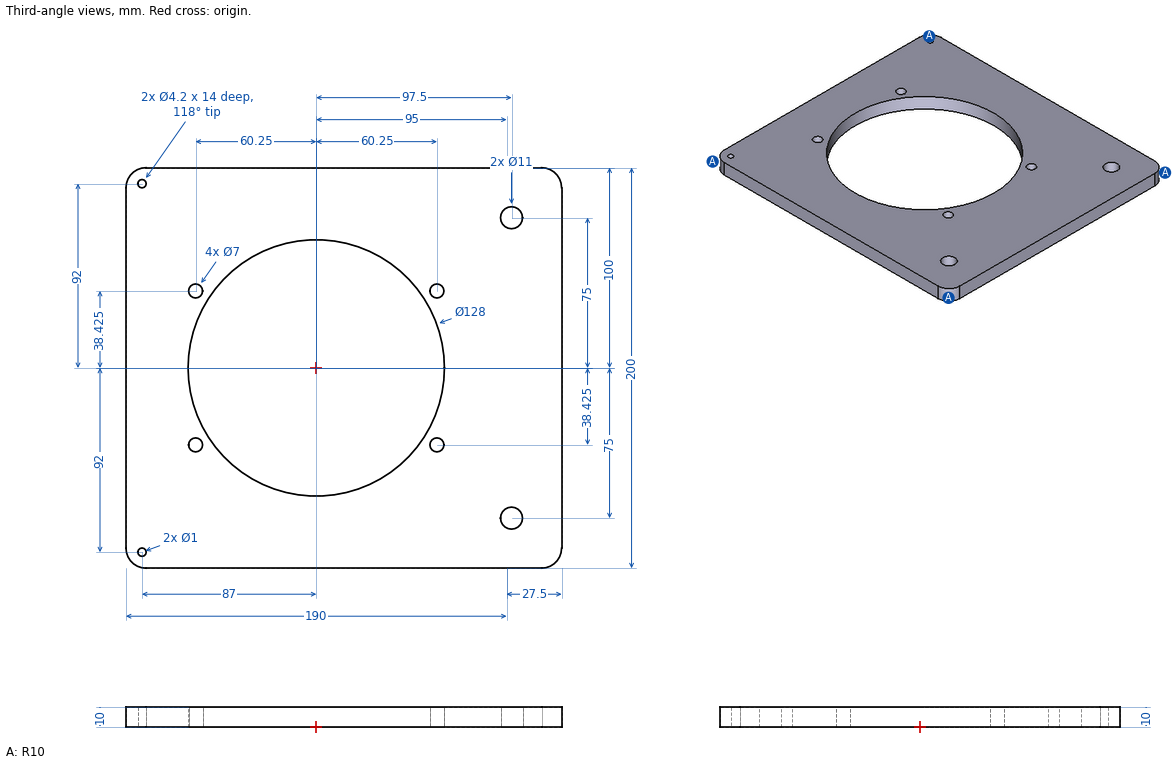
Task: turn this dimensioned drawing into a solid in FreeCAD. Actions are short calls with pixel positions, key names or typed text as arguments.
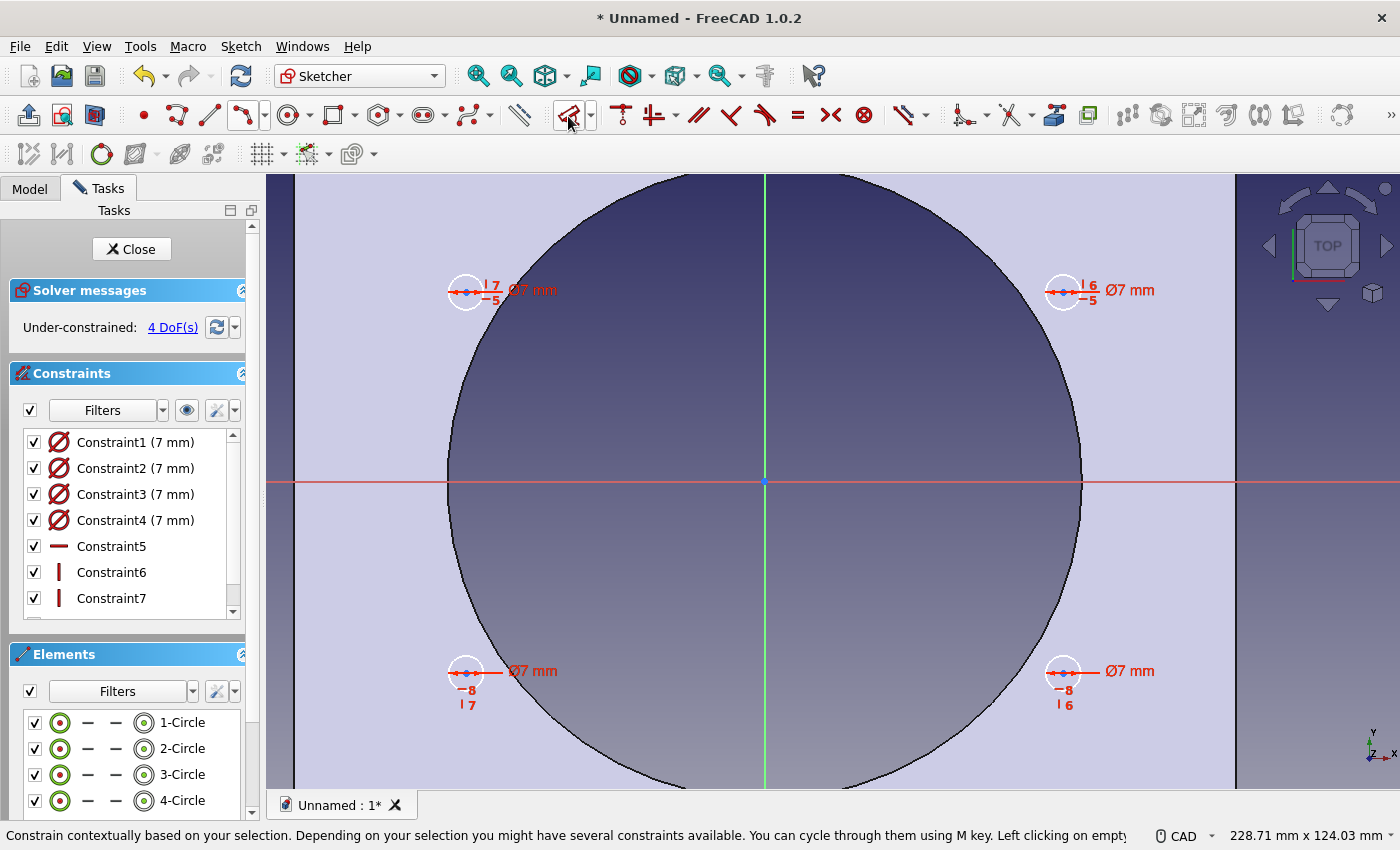
click(466, 292)
click(615, 258)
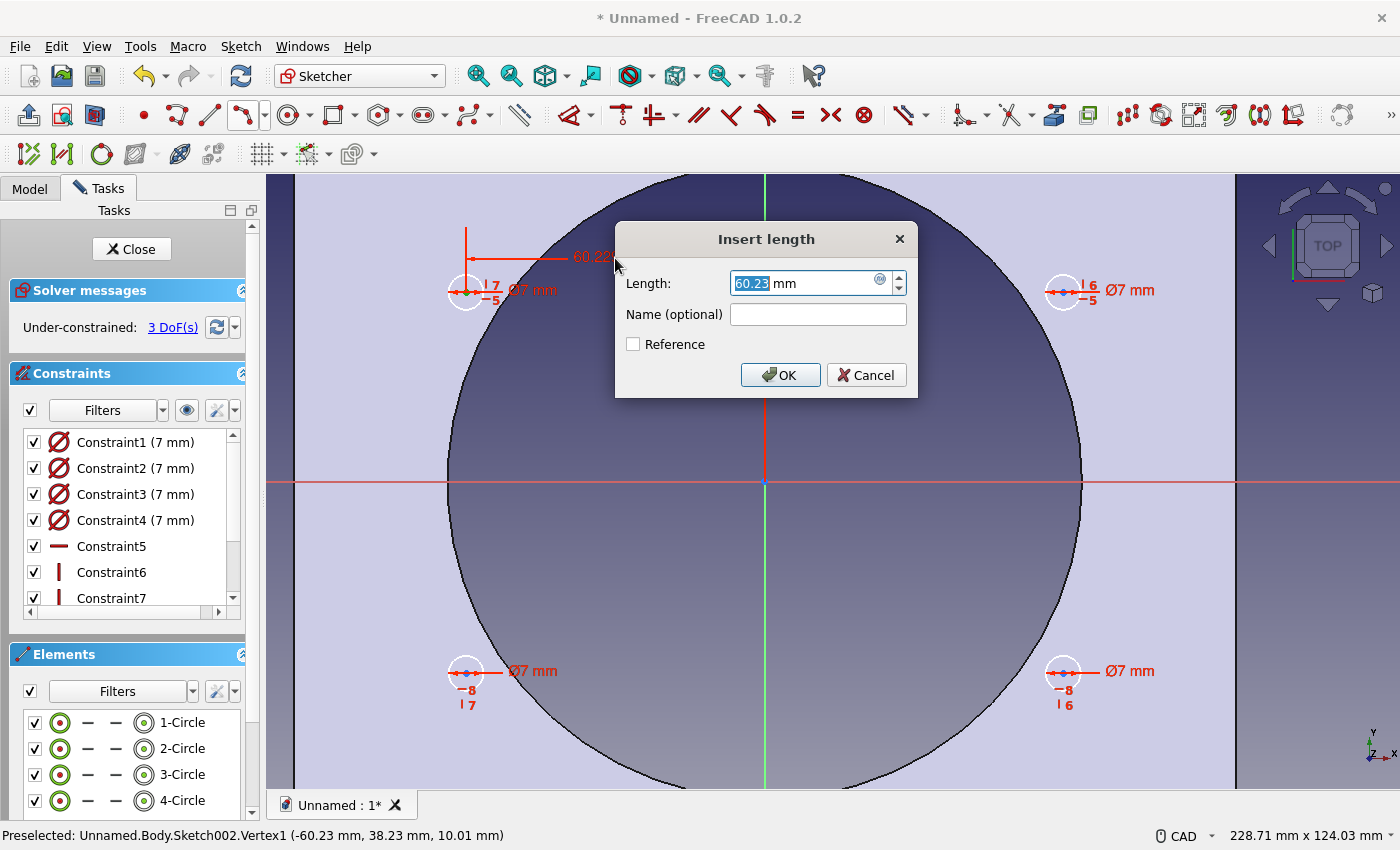
text(60.25)
key(Return)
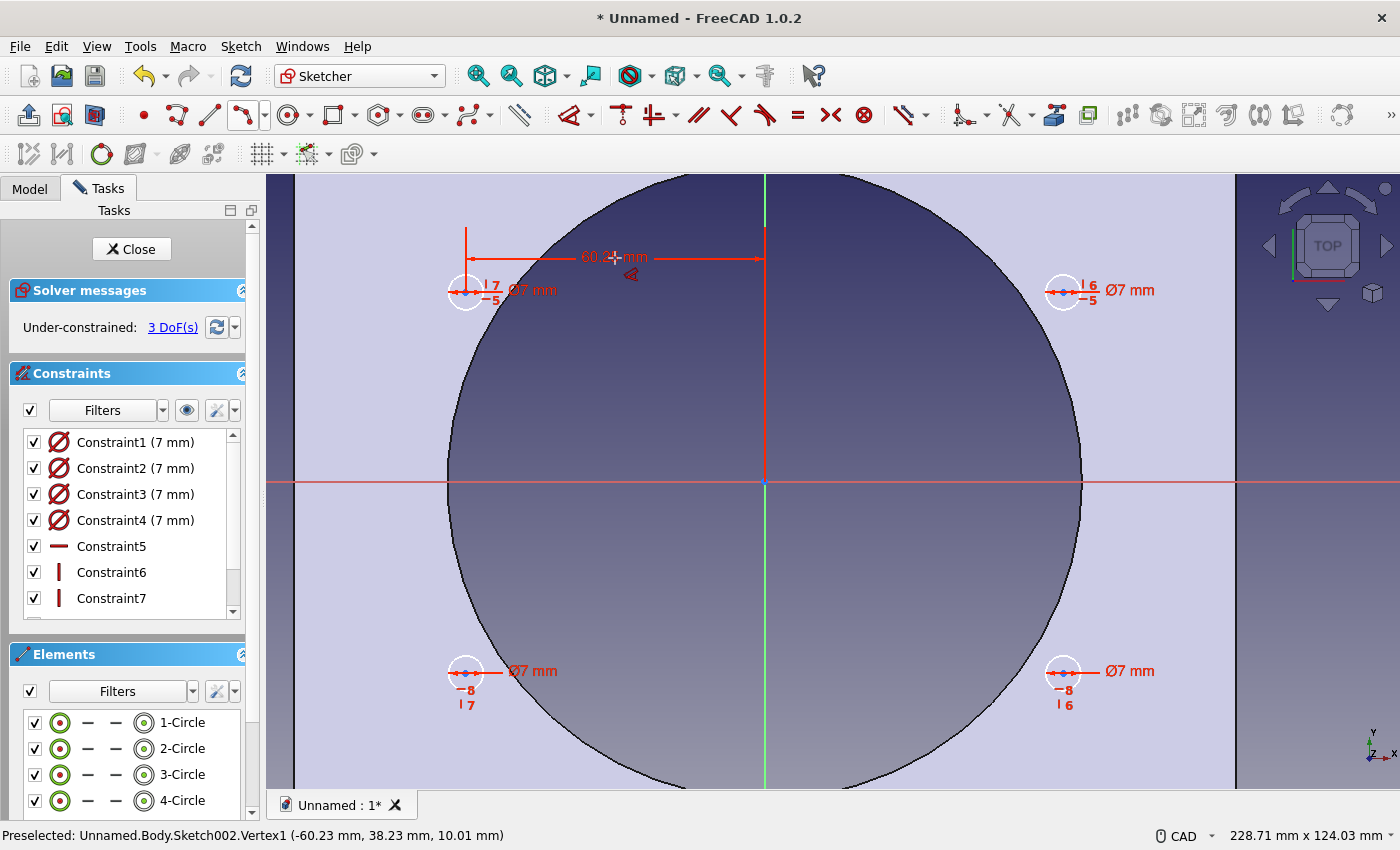
click(1063, 292)
click(914, 258)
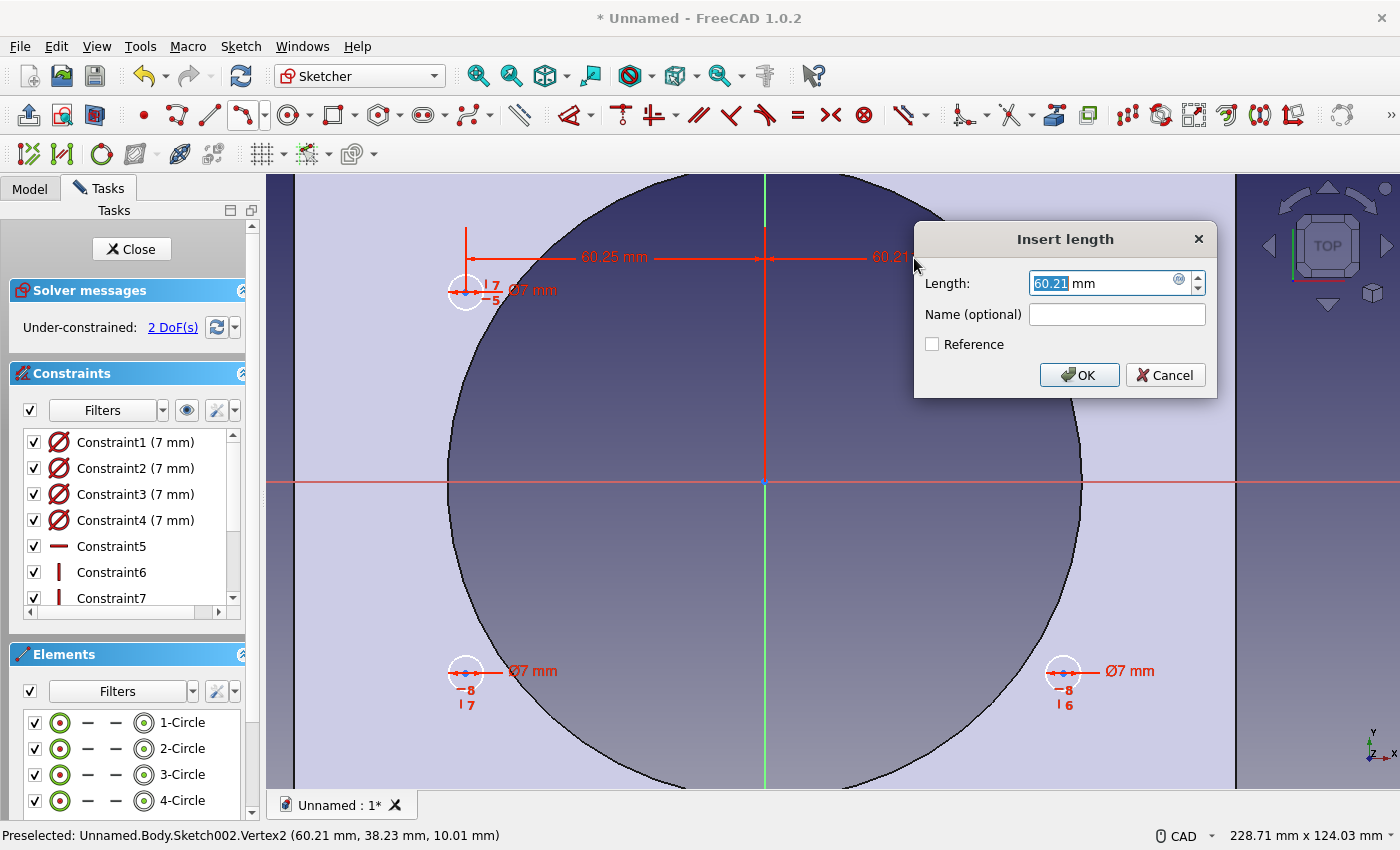
text(60.25)
key(Return)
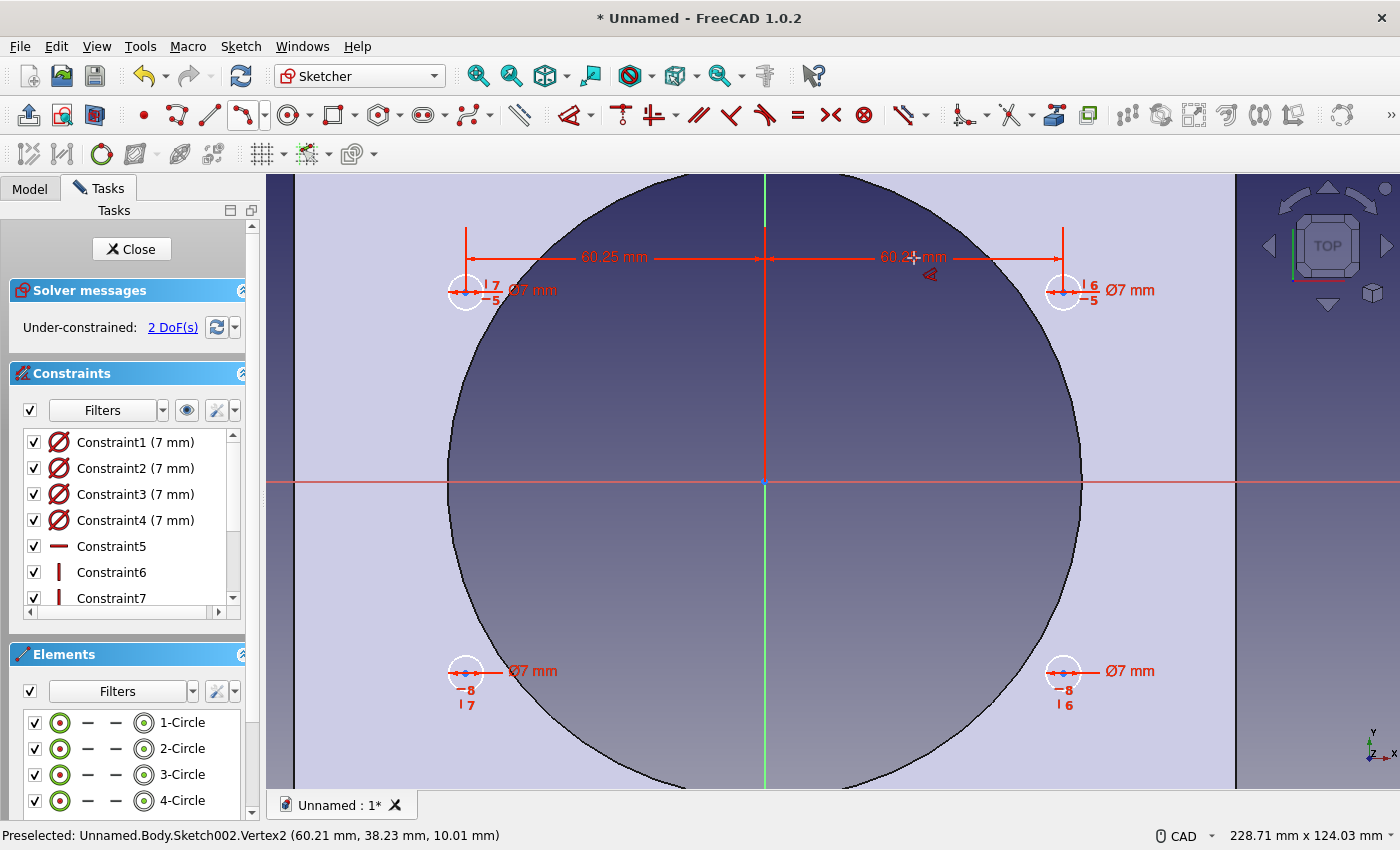
click(466, 292)
click(432, 387)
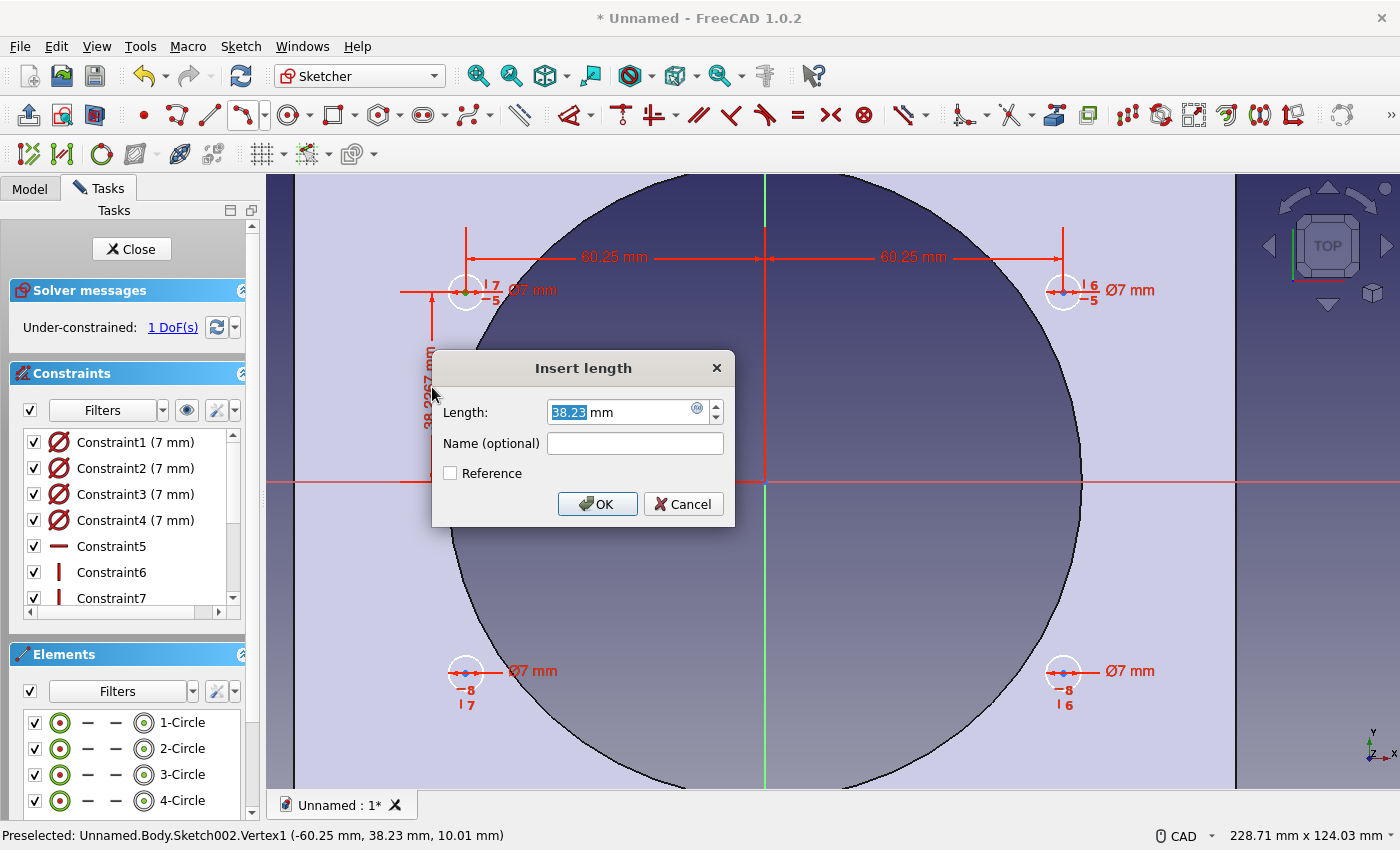
text(38.425)
key(Return)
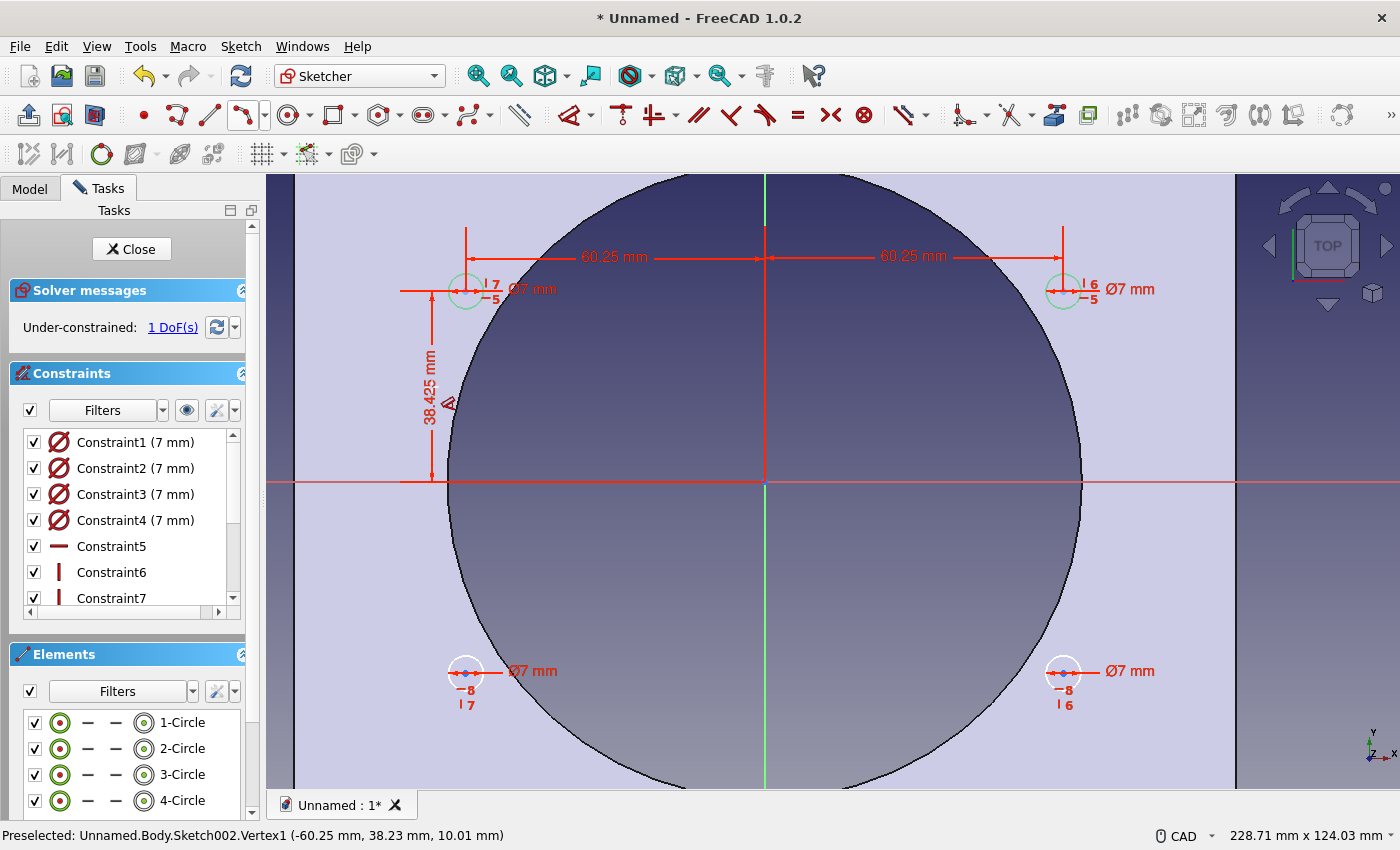
click(1063, 673)
click(1097, 578)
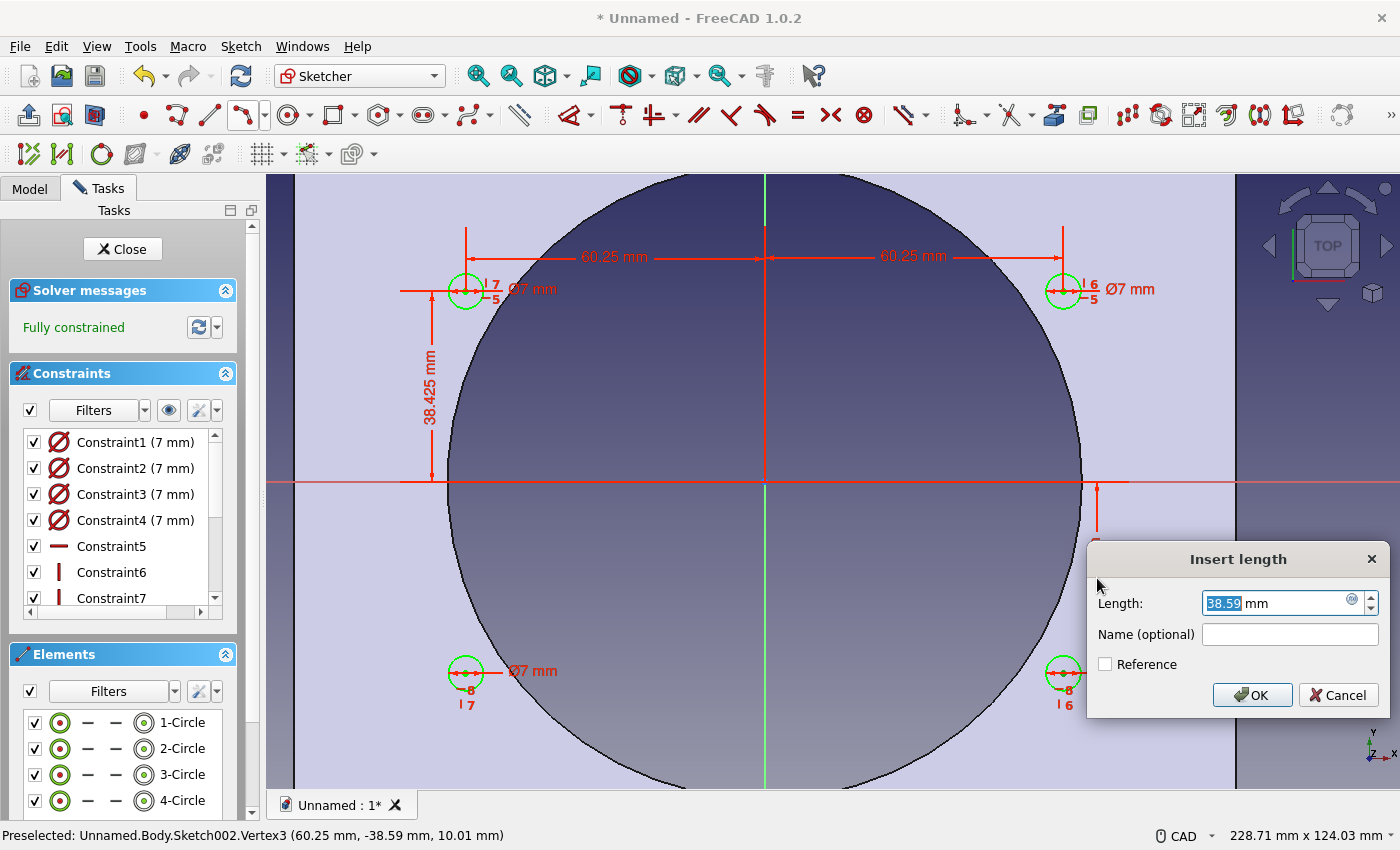
text(38.425)
key(Return)
key(Escape)